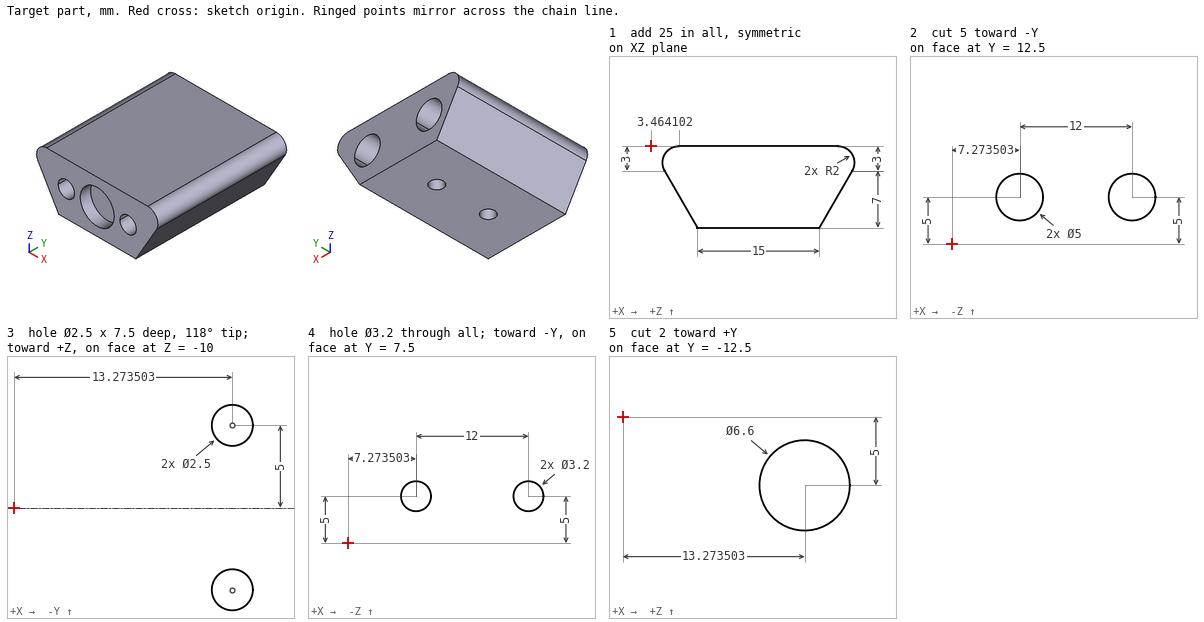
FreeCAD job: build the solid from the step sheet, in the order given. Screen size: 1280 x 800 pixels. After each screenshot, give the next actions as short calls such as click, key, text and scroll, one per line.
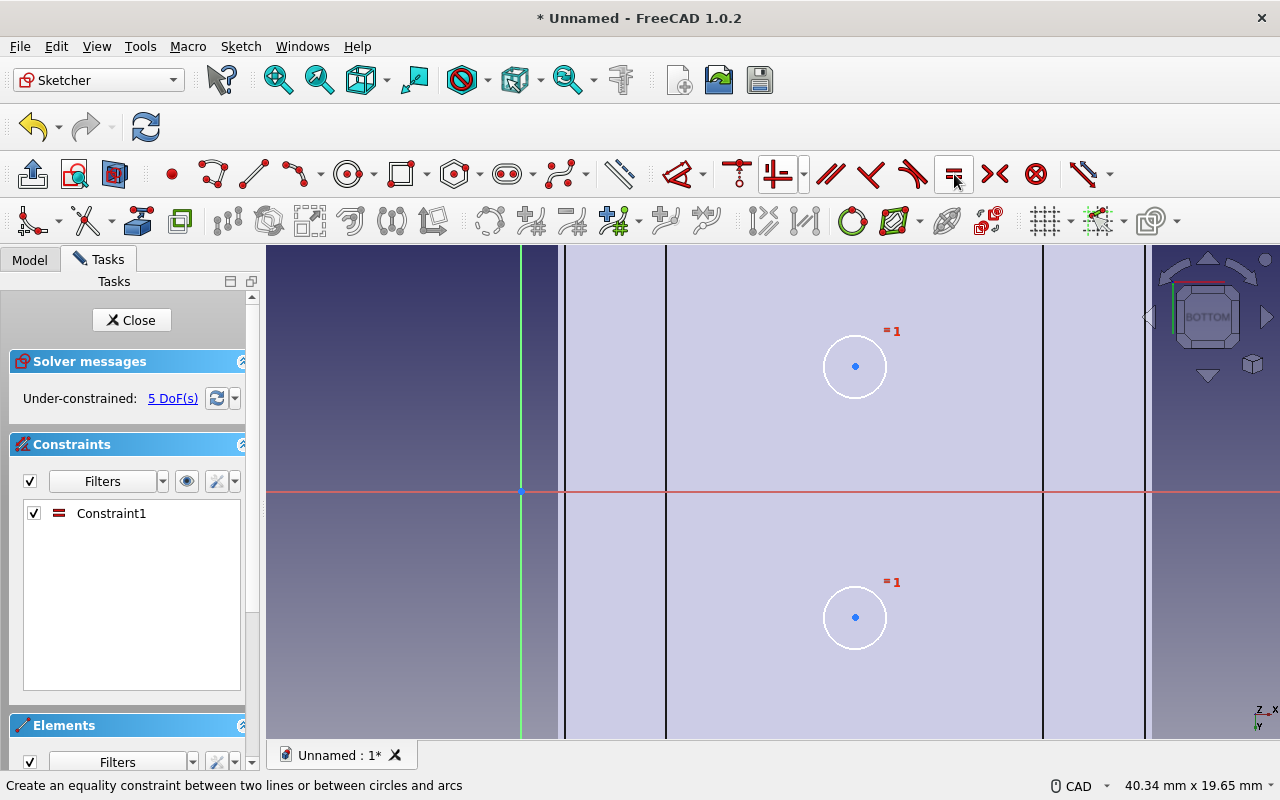
click(855, 367)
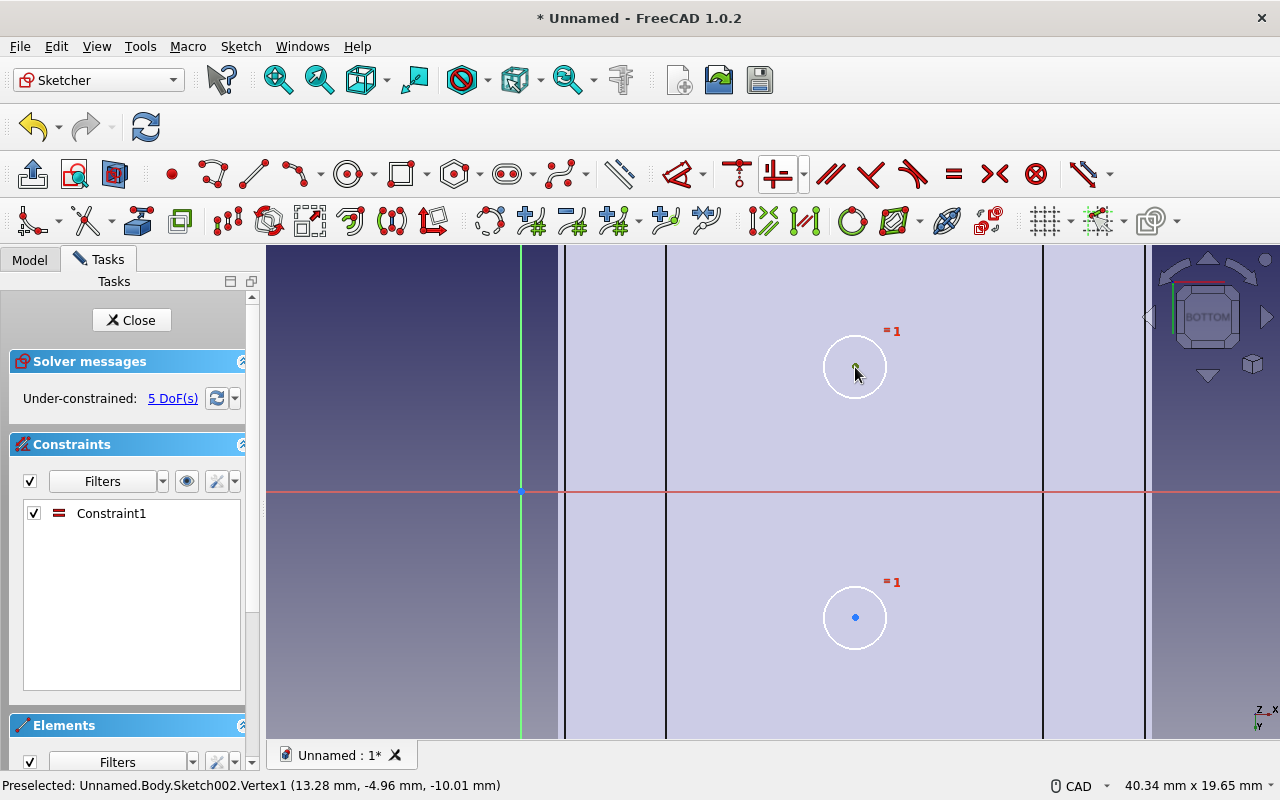
click(855, 618)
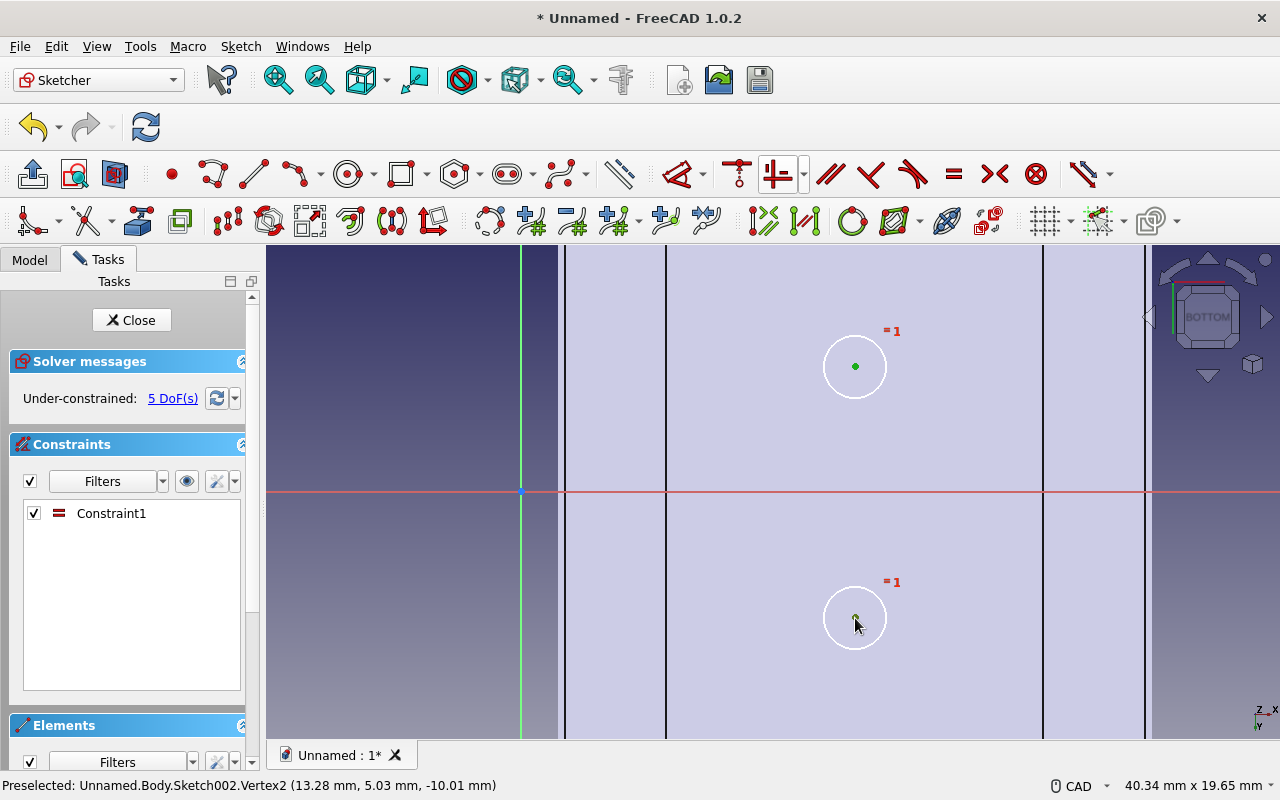
click(353, 492)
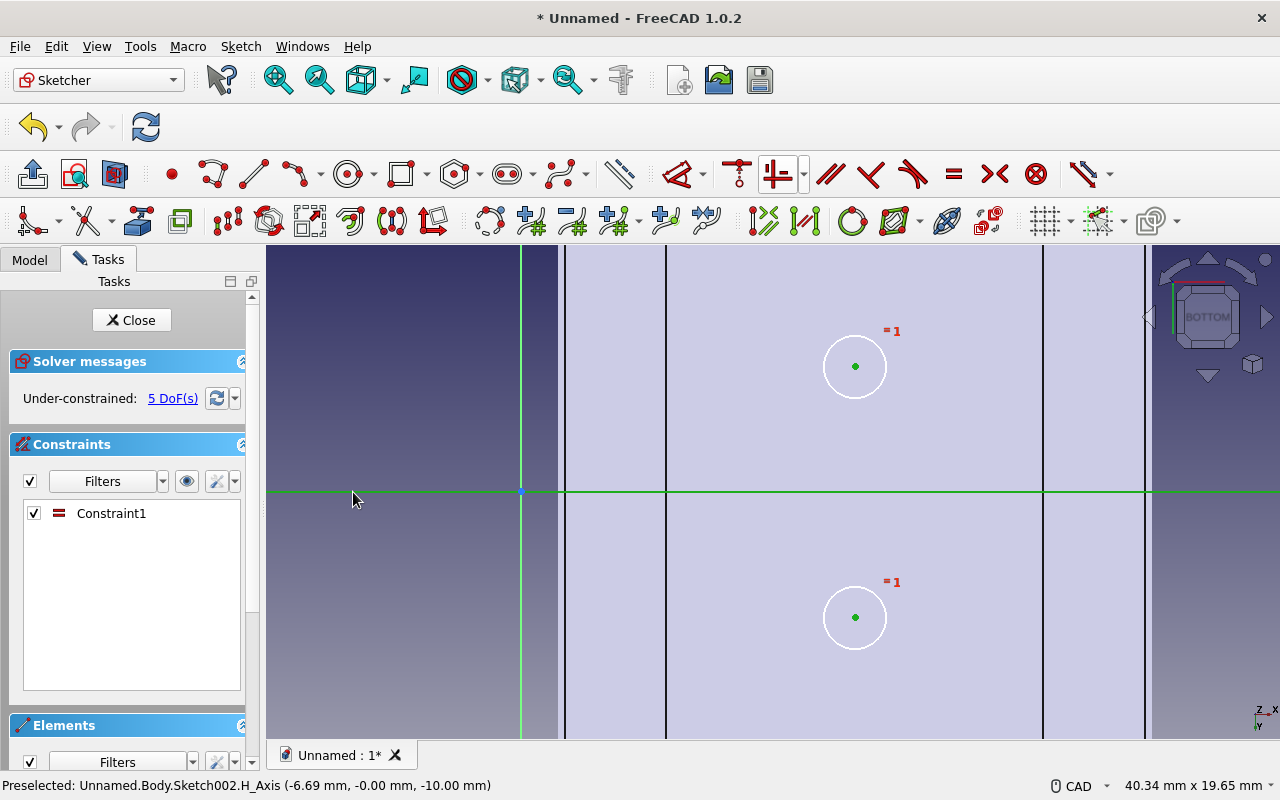
click(995, 174)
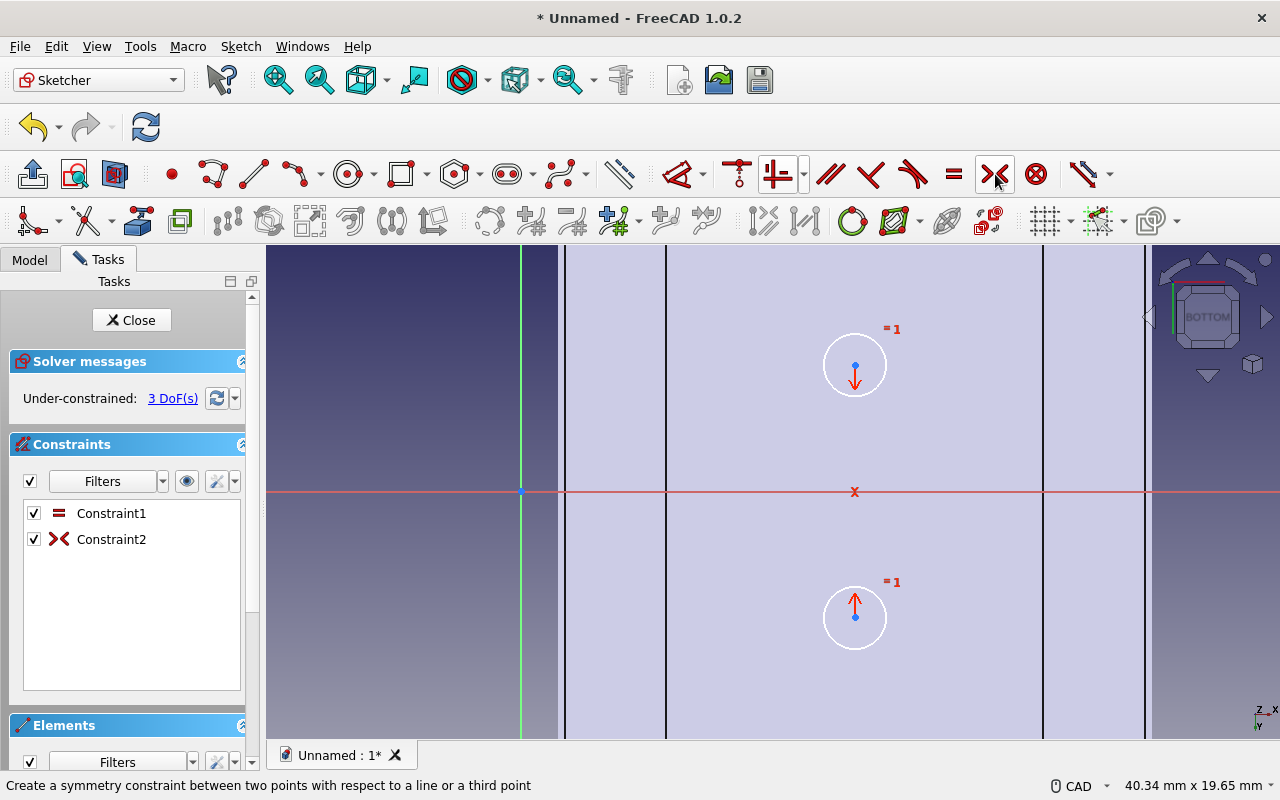
click(676, 174)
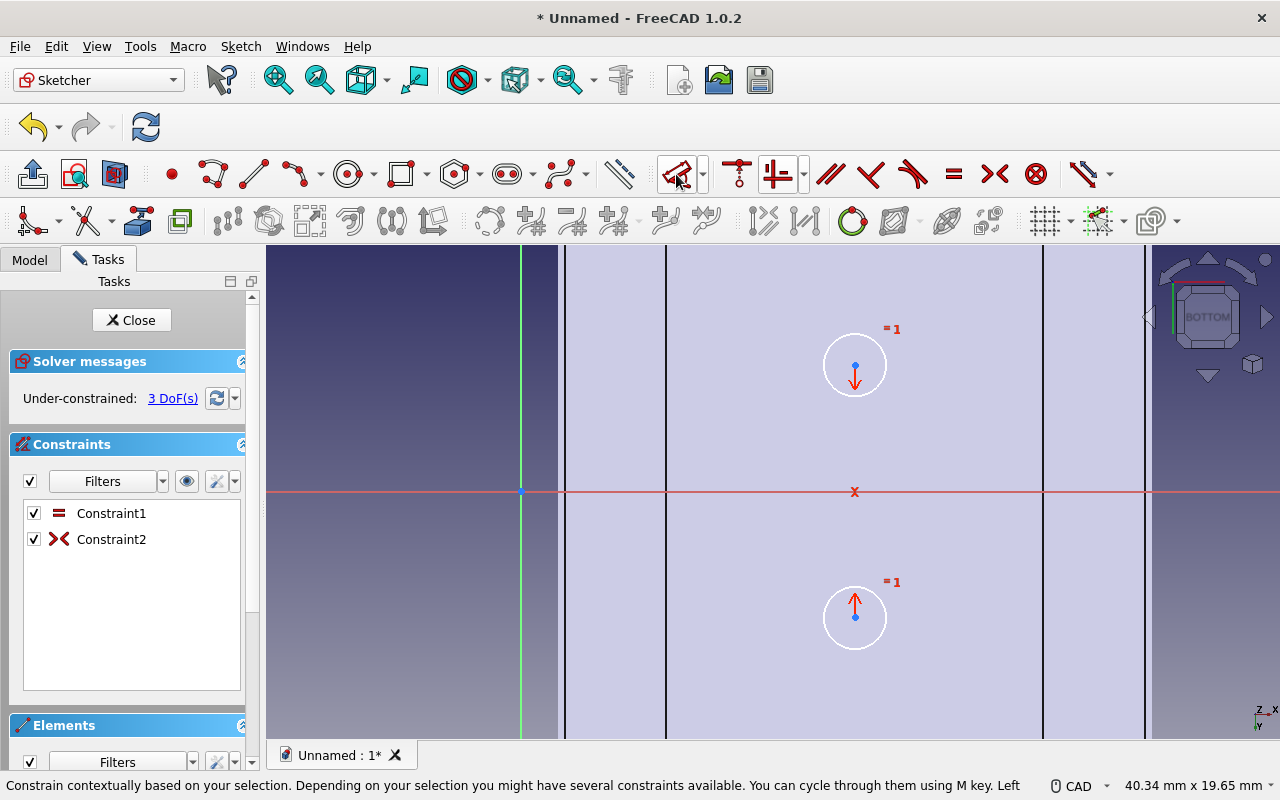
click(877, 343)
click(900, 320)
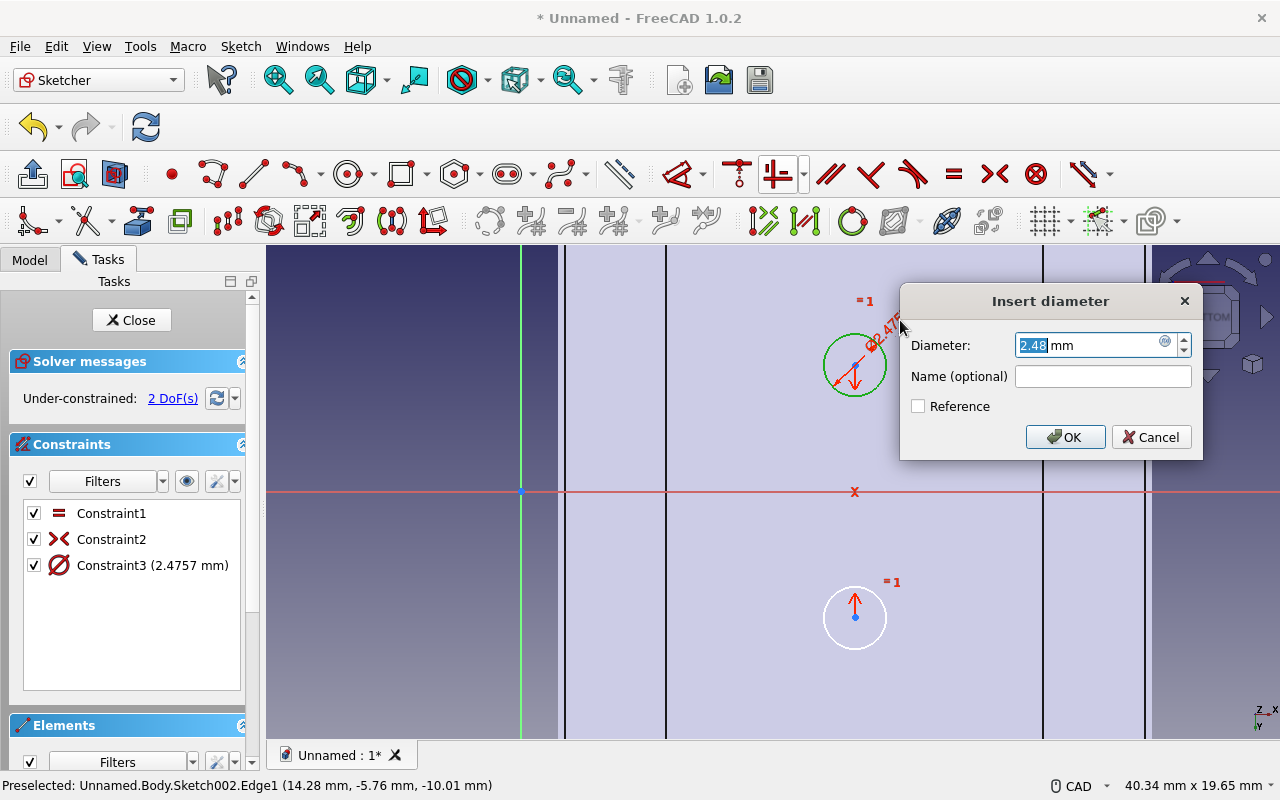
text(2.5)
key(Return)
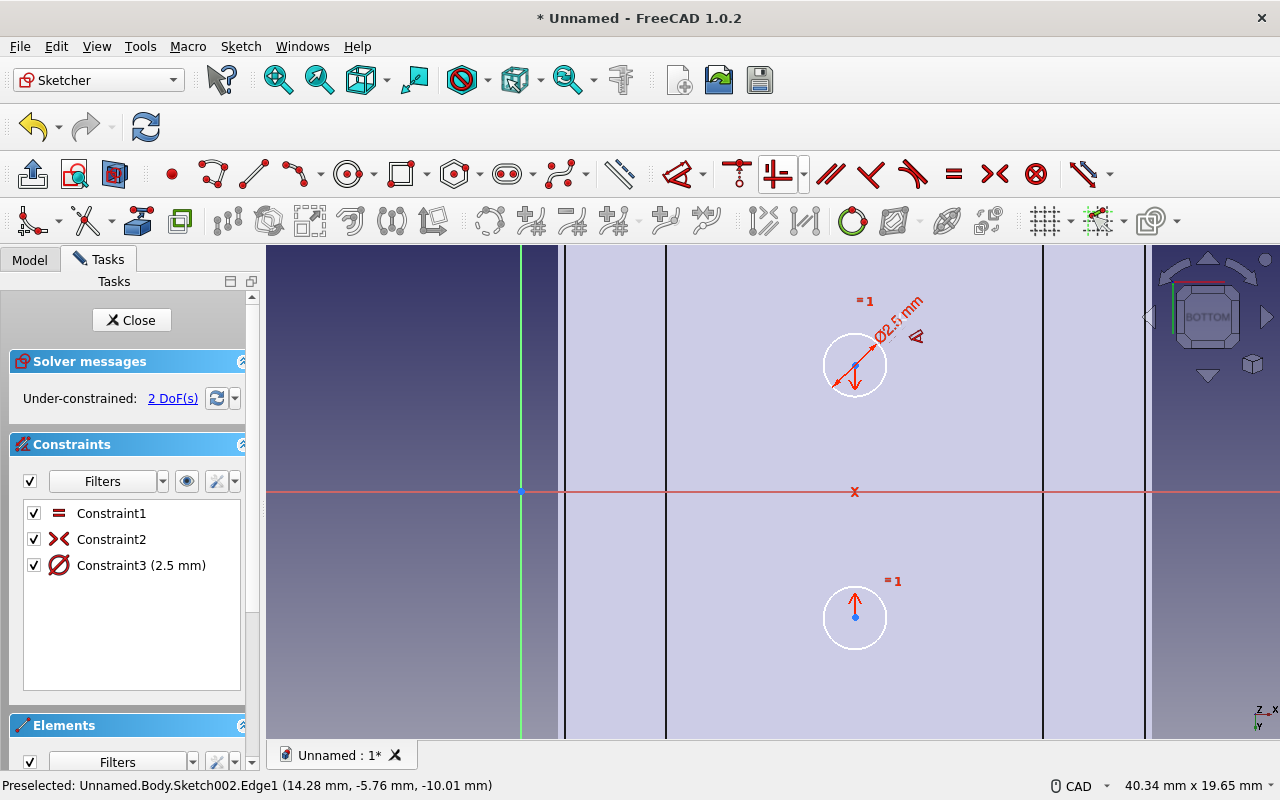
click(855, 365)
click(487, 428)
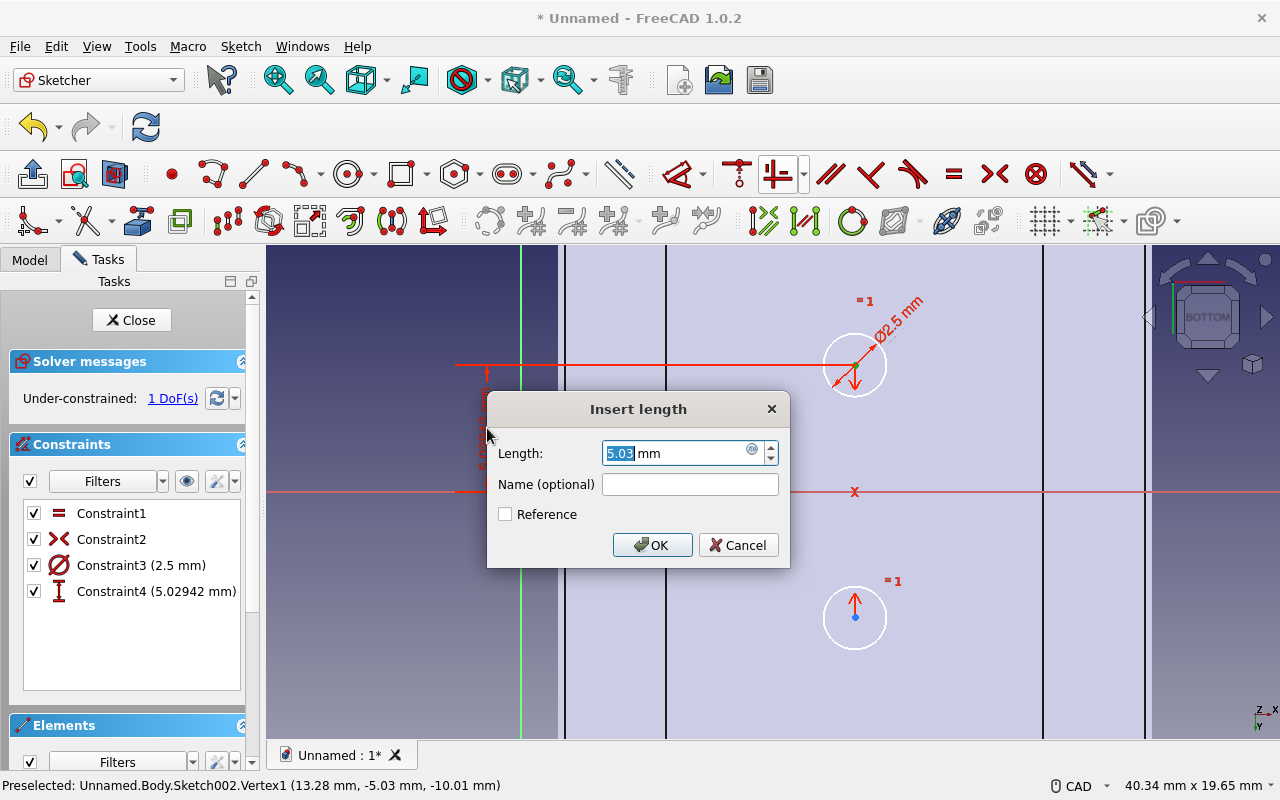
text(5)
key(Return)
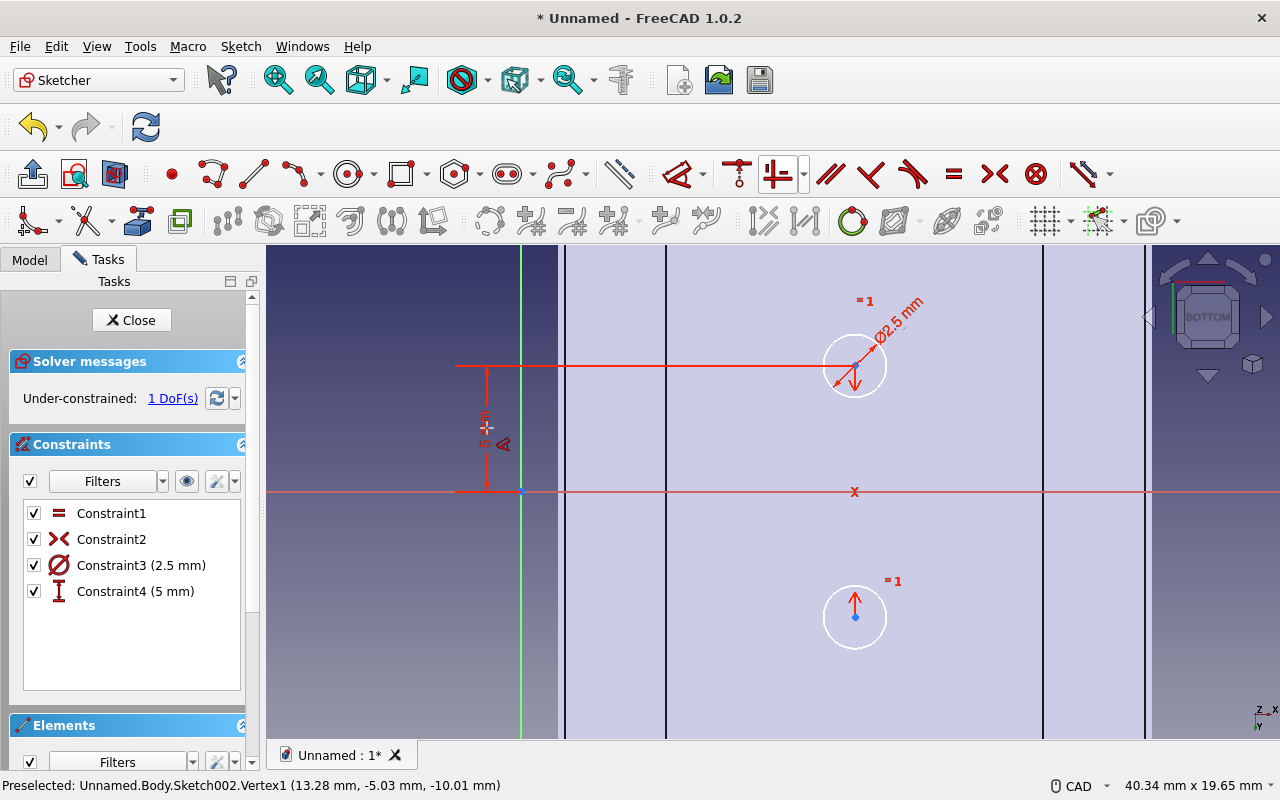
click(855, 366)
click(688, 332)